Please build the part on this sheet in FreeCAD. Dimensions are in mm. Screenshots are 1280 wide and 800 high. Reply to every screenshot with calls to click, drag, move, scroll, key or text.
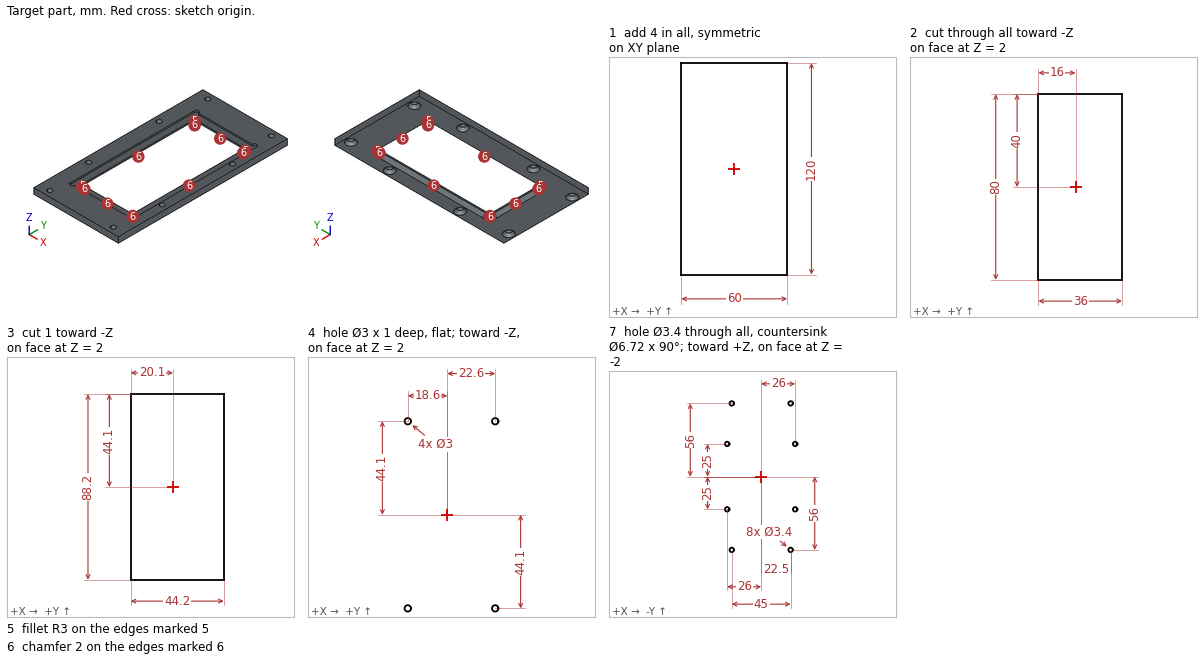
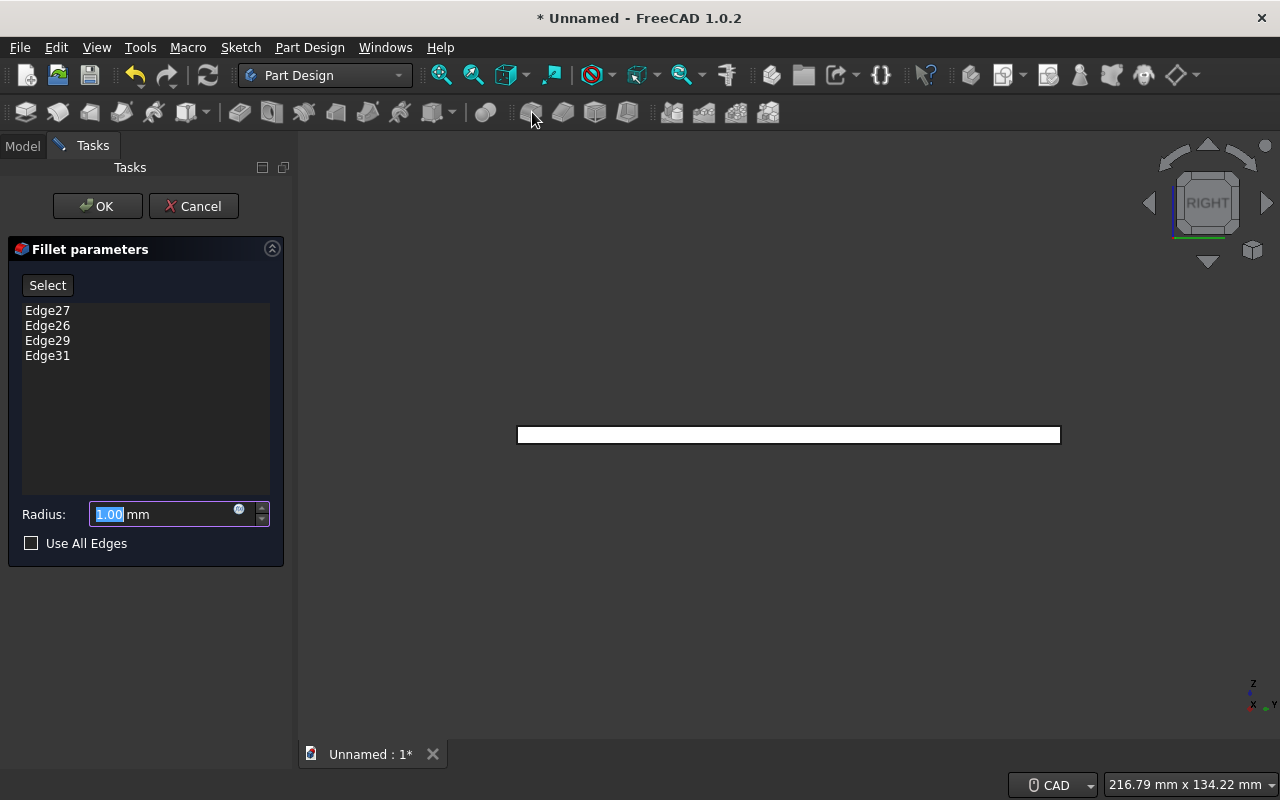
text(3)
key(Tab)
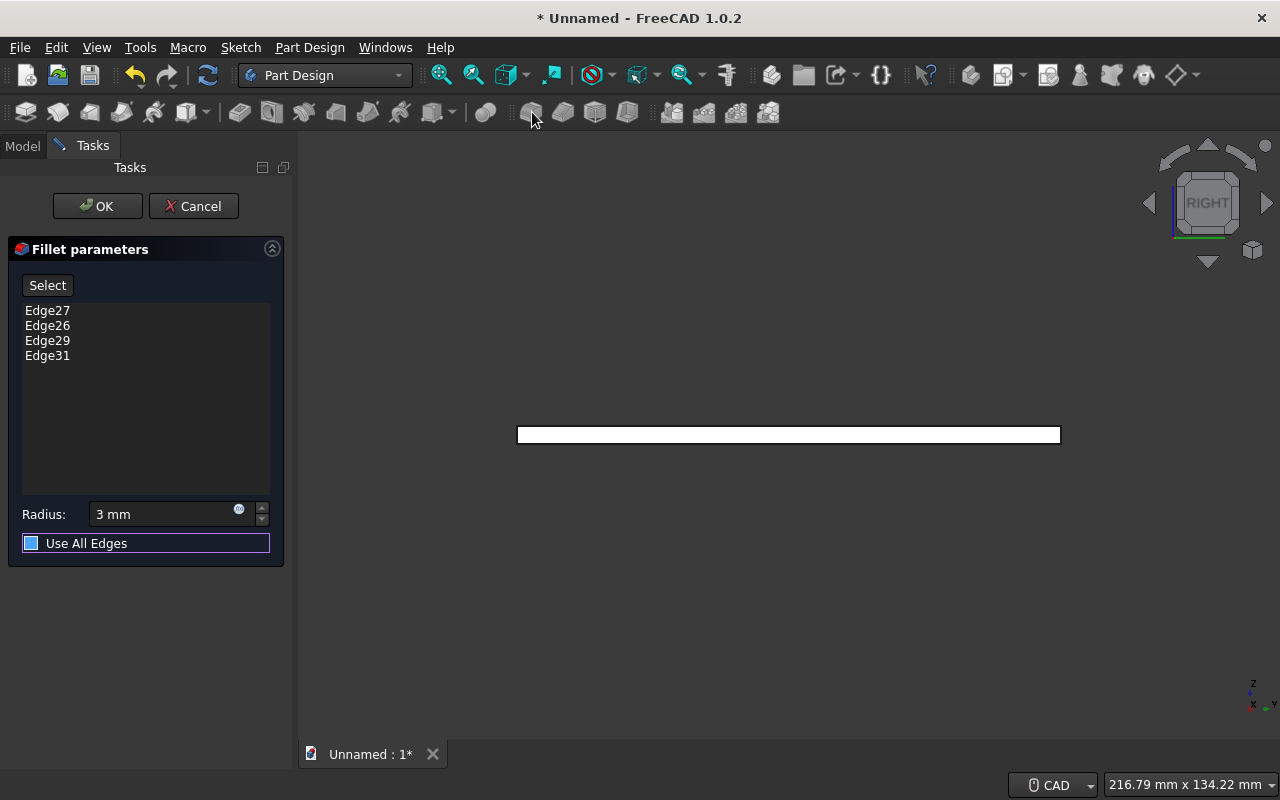
click(98, 206)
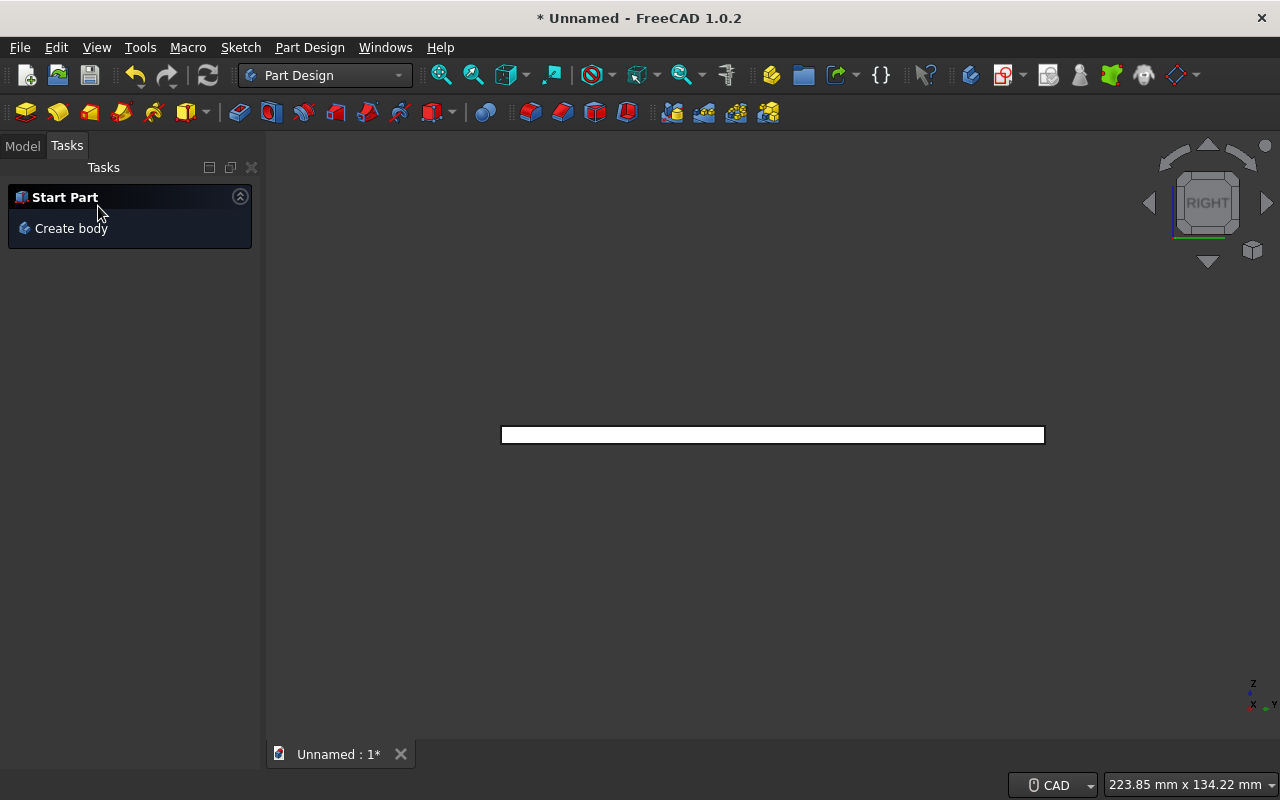
key(0)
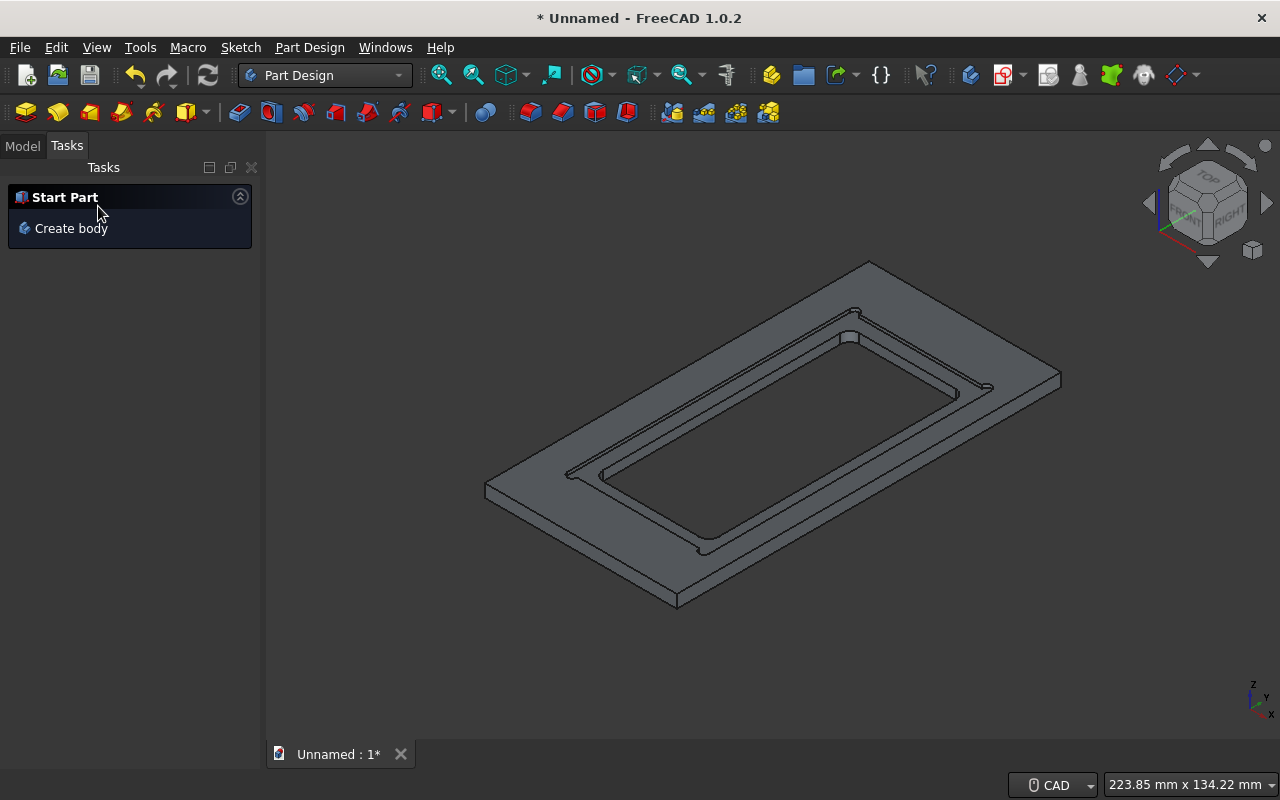
key(2)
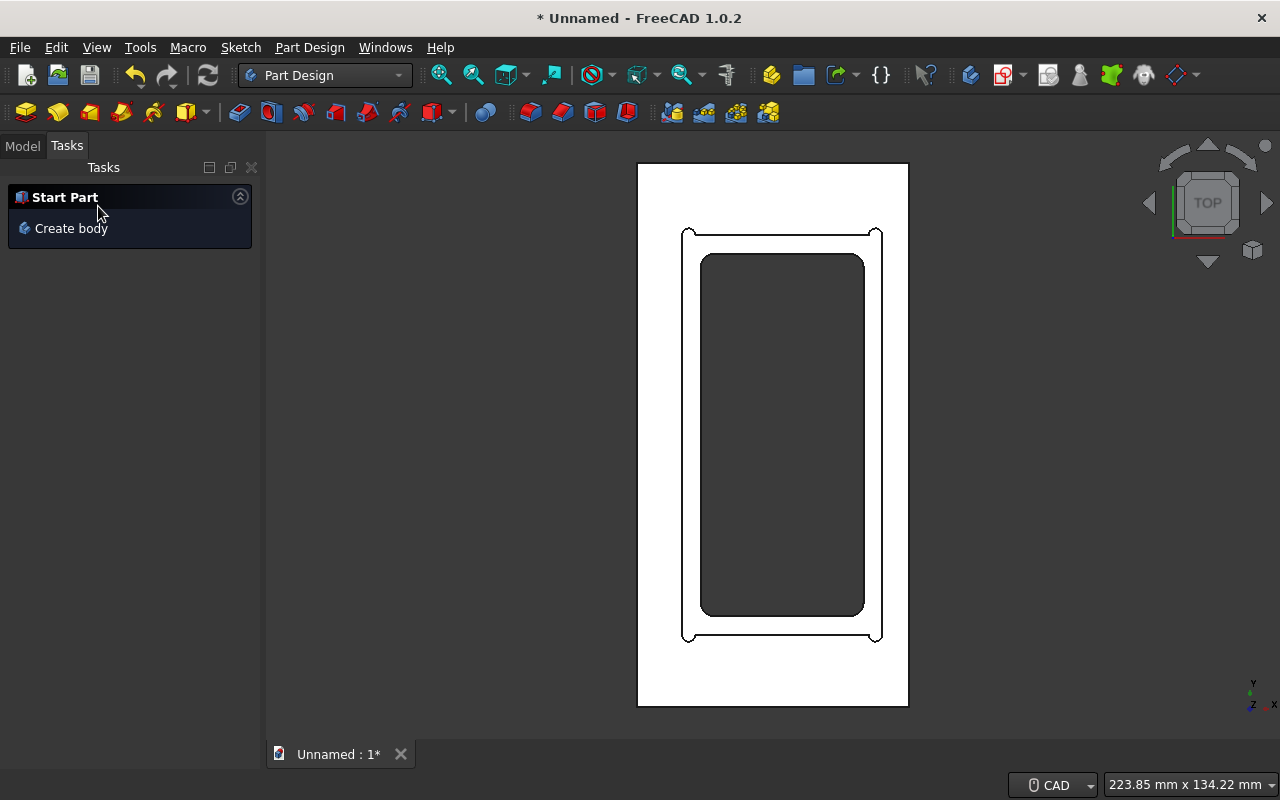
key(1)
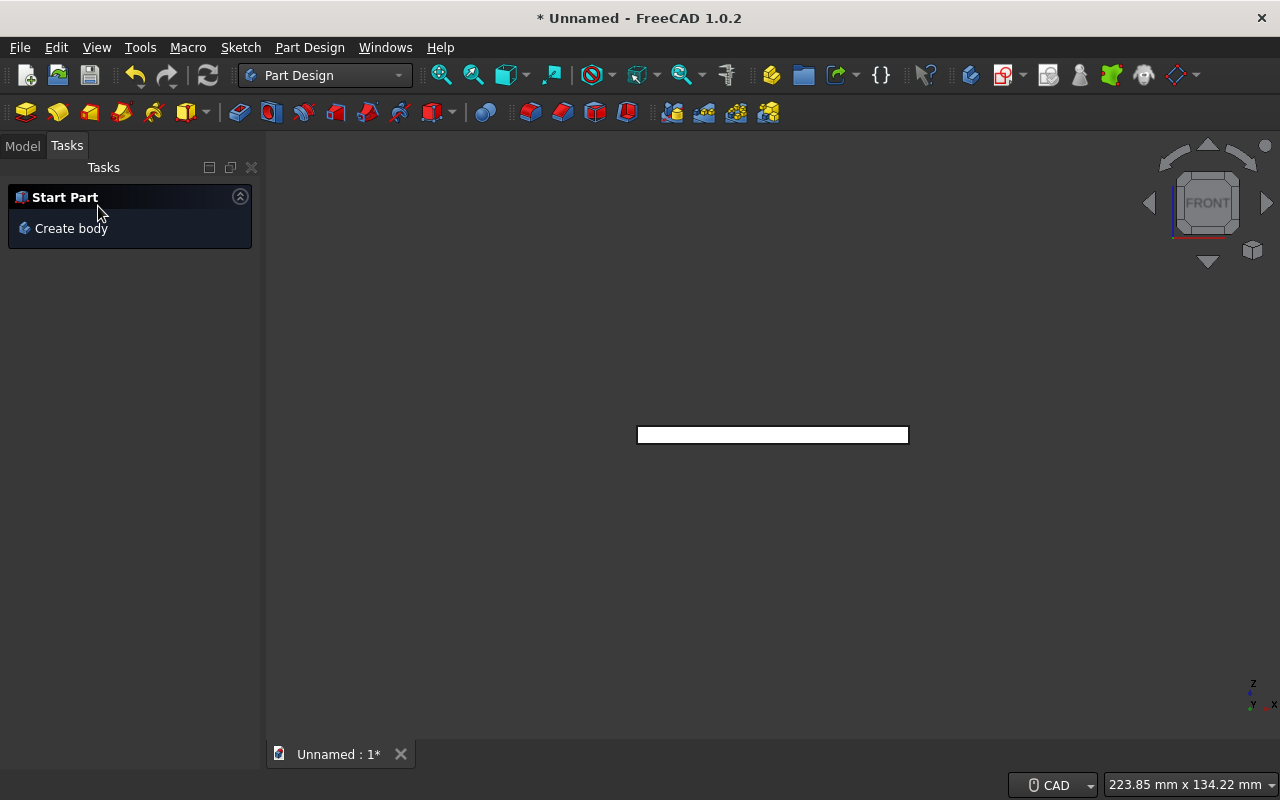
click(442, 76)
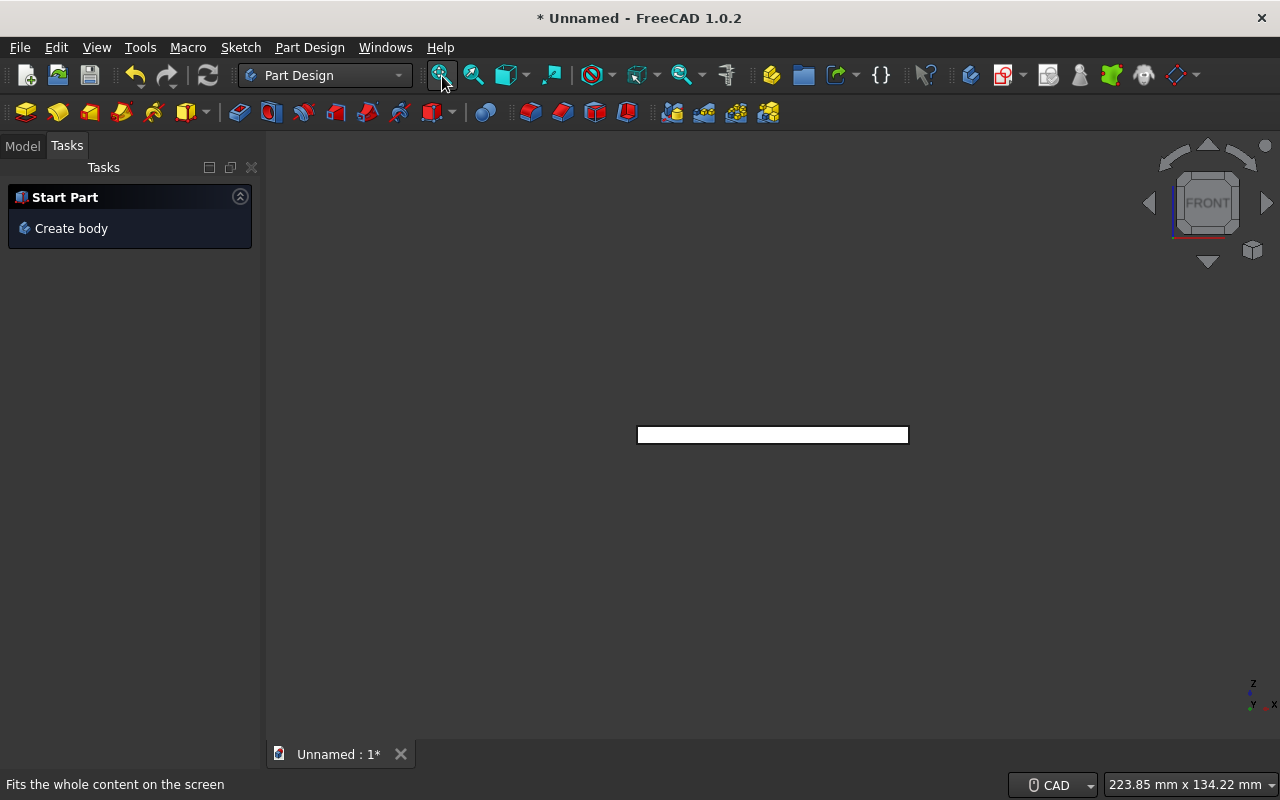
key(3)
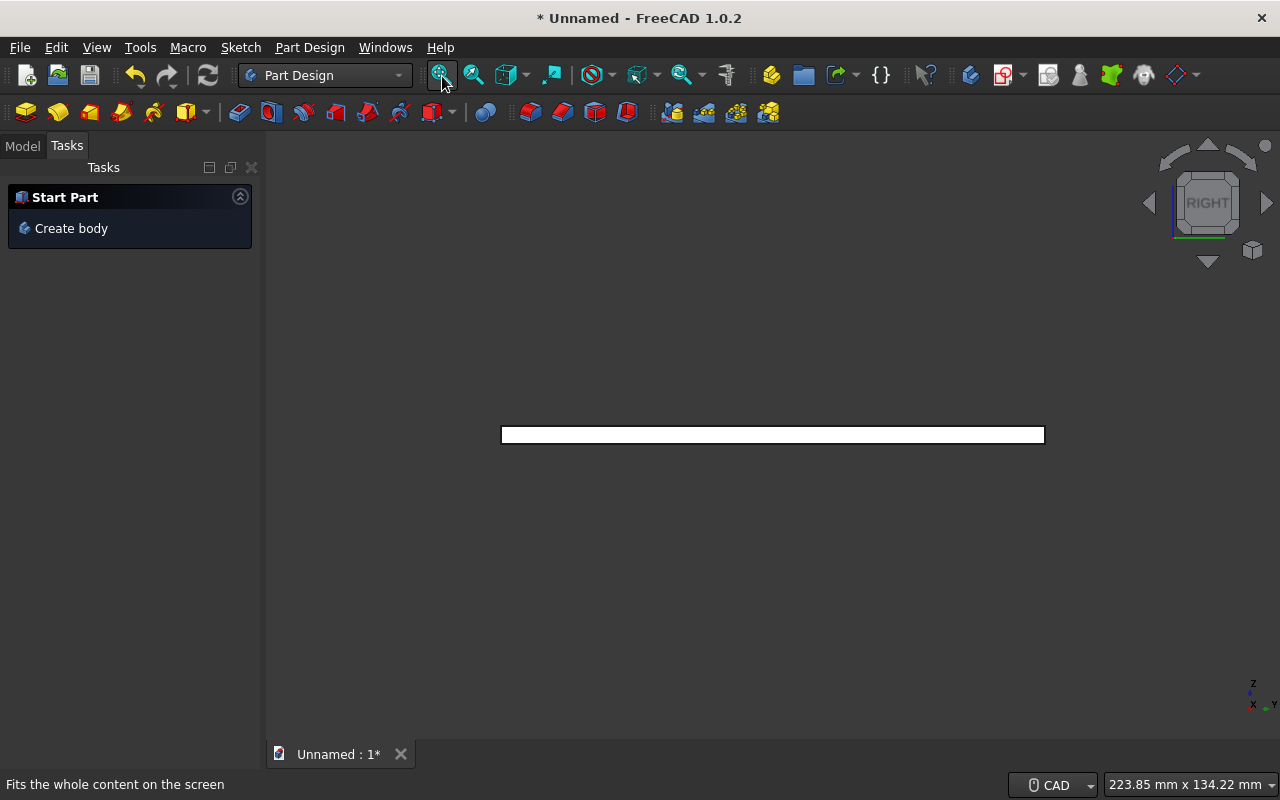
key(5)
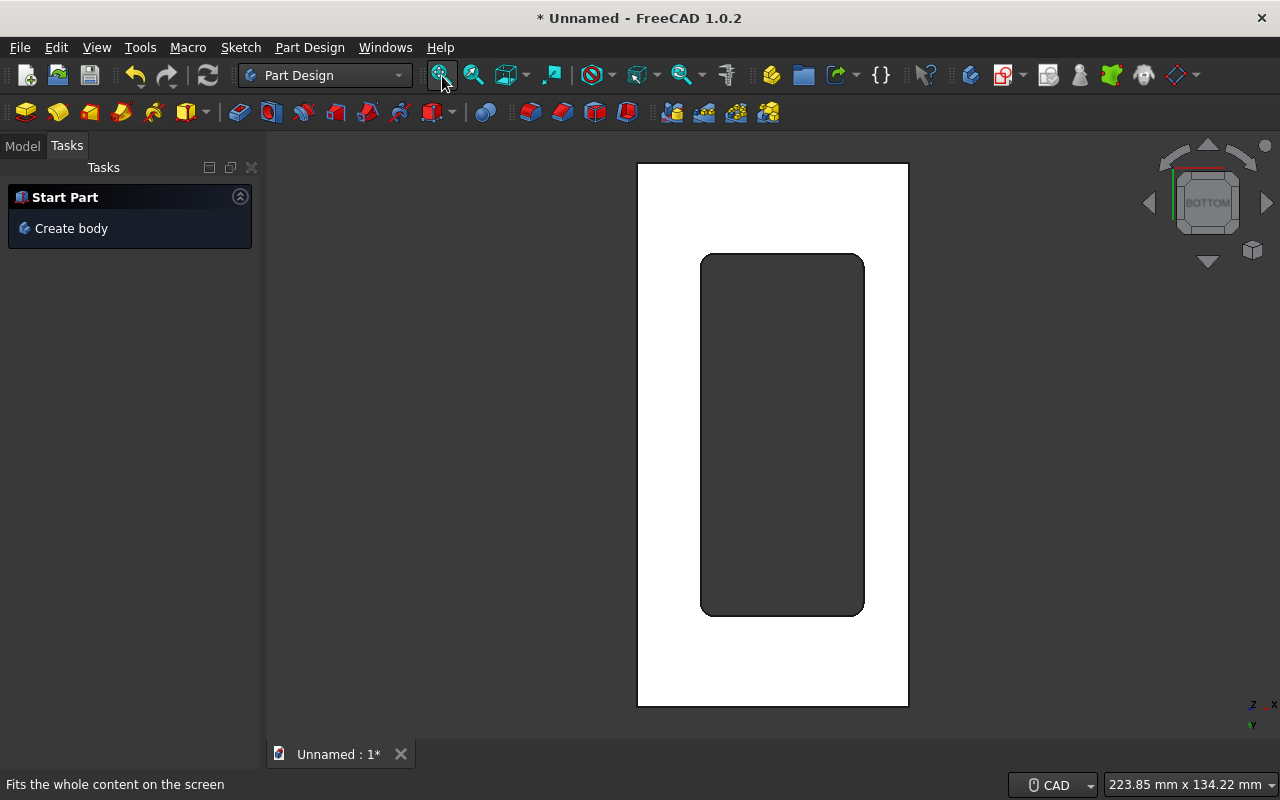
click(864, 434)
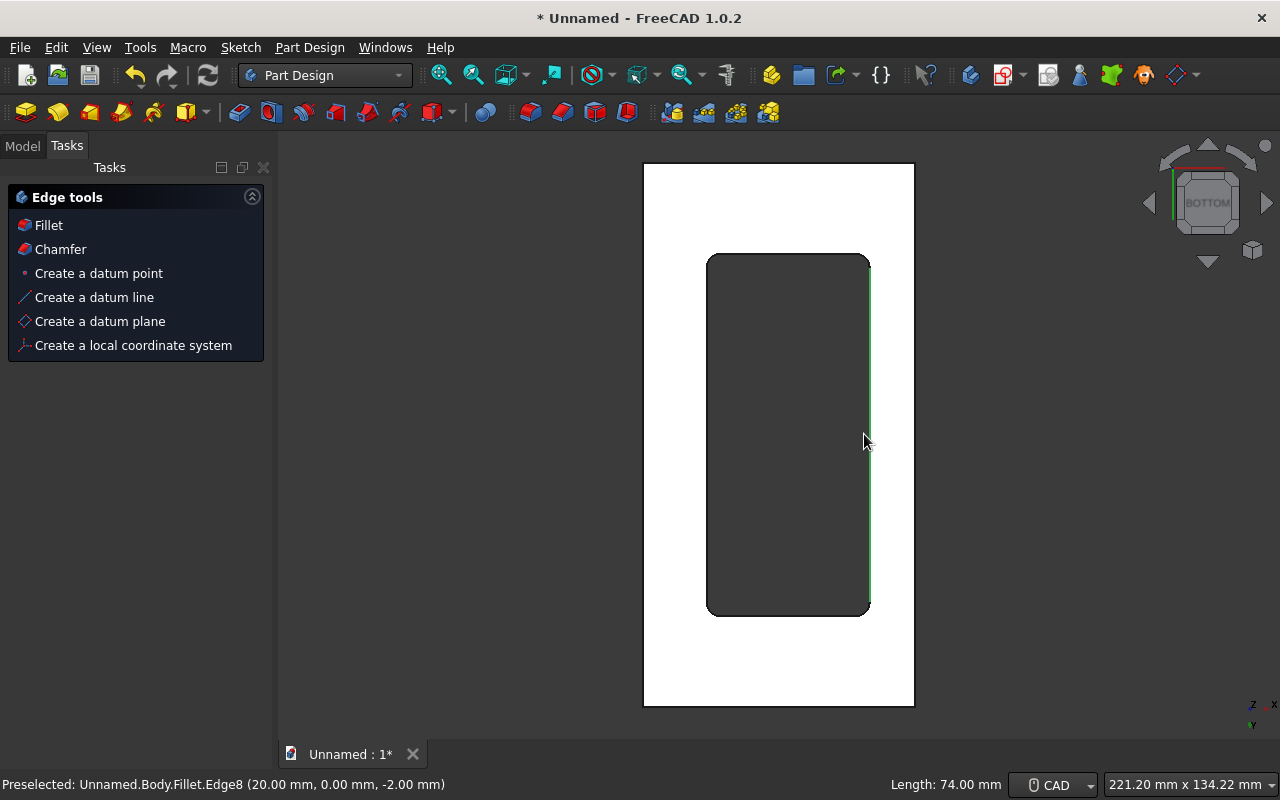
click(788, 253, ctrl)